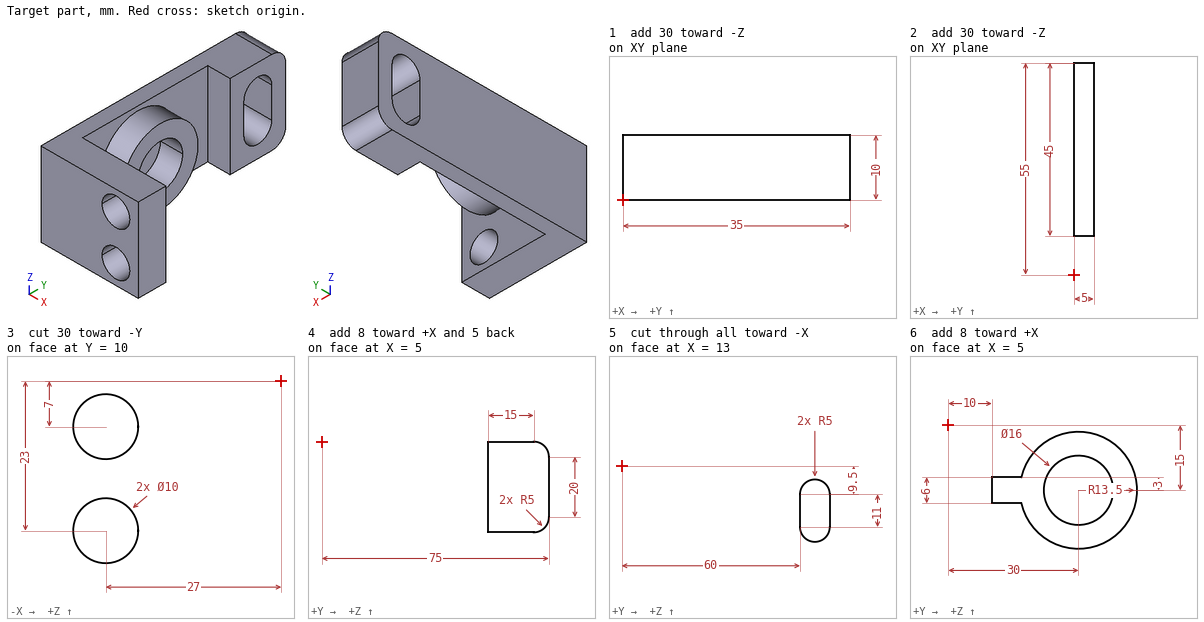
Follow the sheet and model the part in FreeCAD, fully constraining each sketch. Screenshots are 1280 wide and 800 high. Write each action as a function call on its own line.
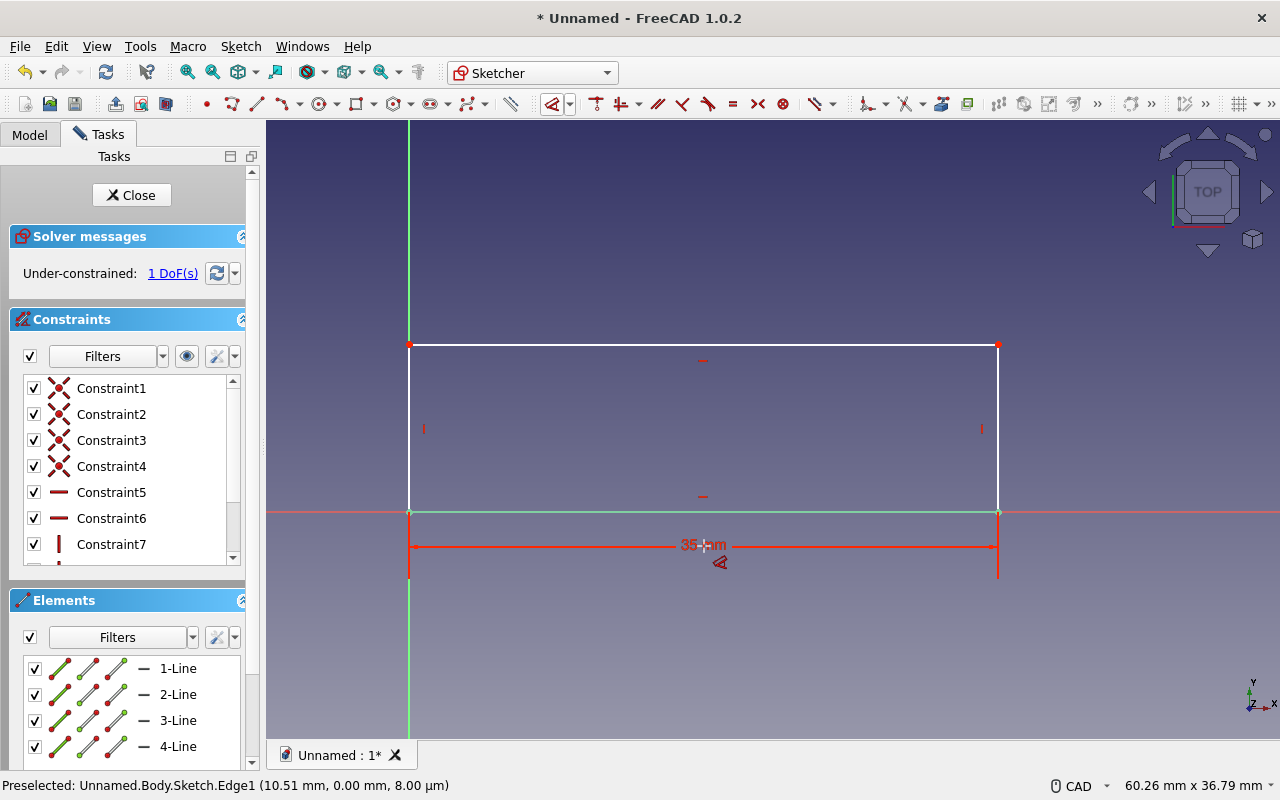
click(998, 462)
click(1032, 429)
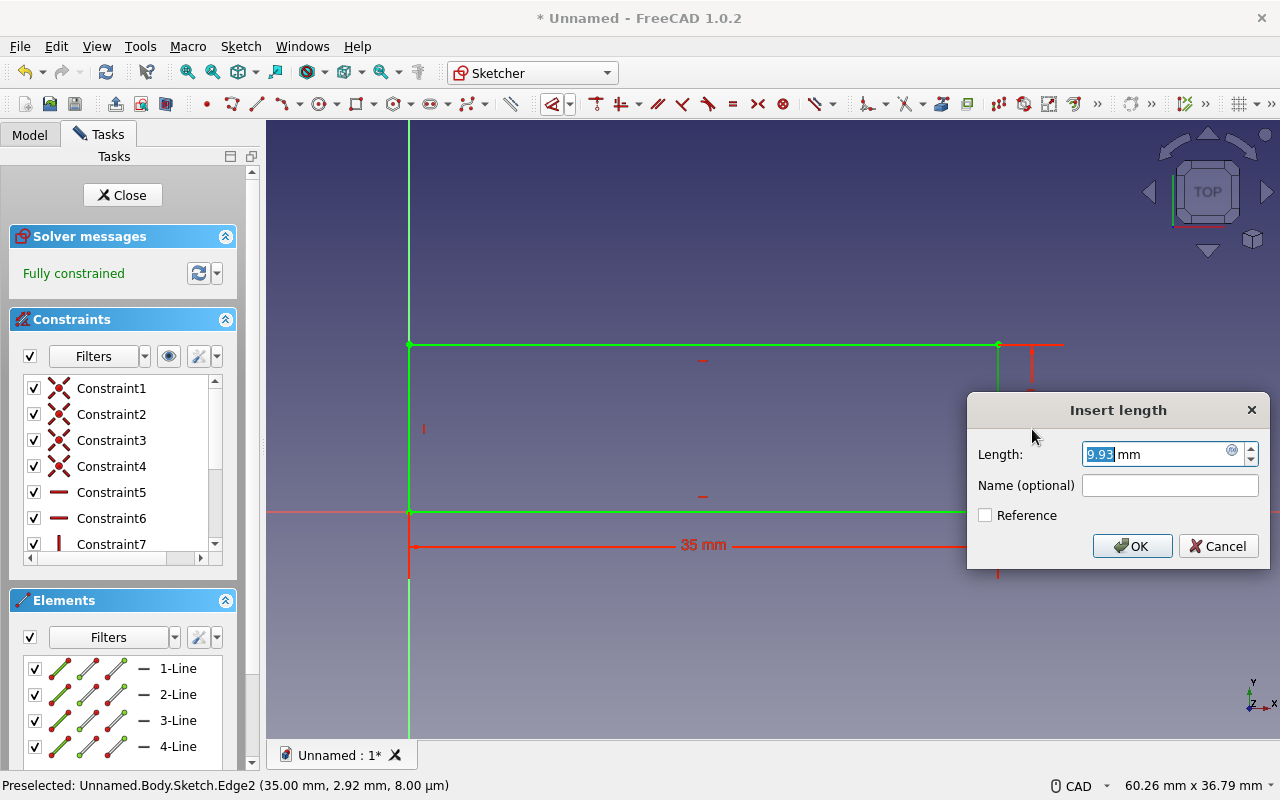
text(10)
key(Return)
key(Escape)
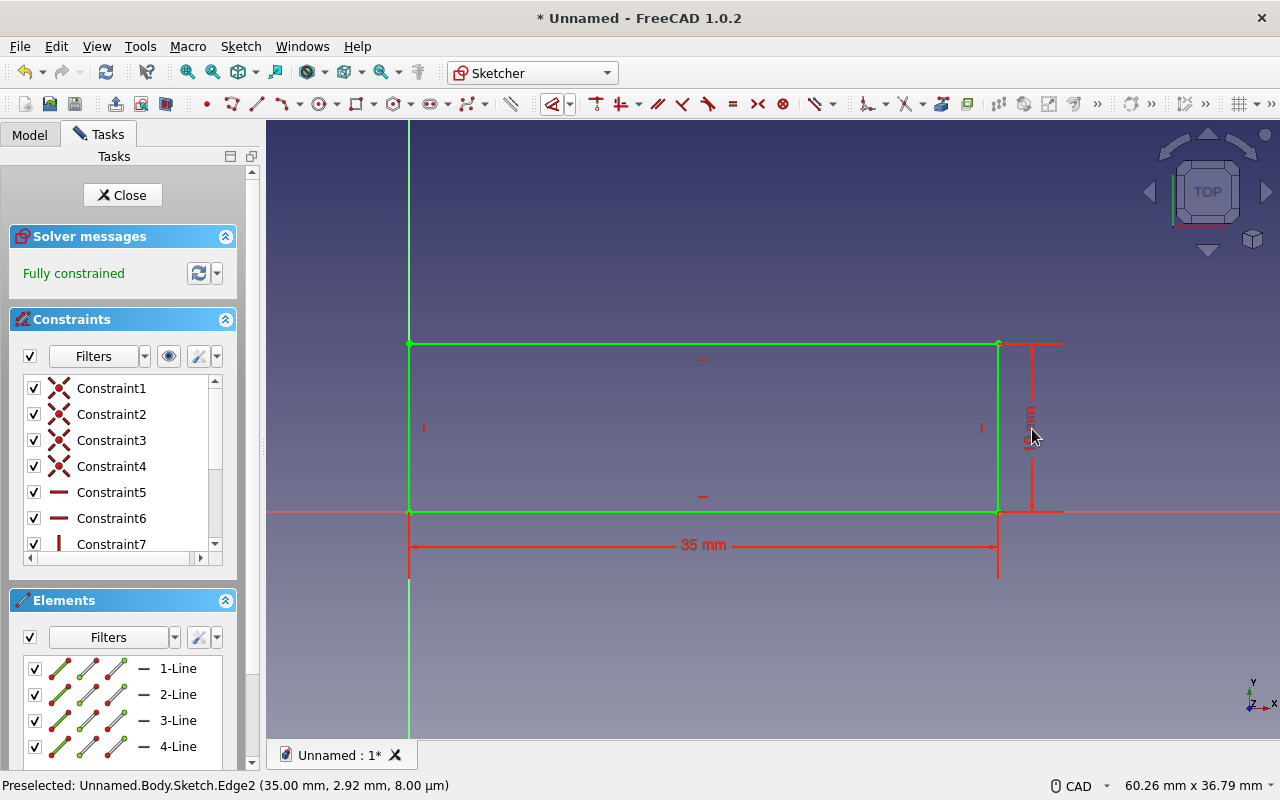
click(123, 195)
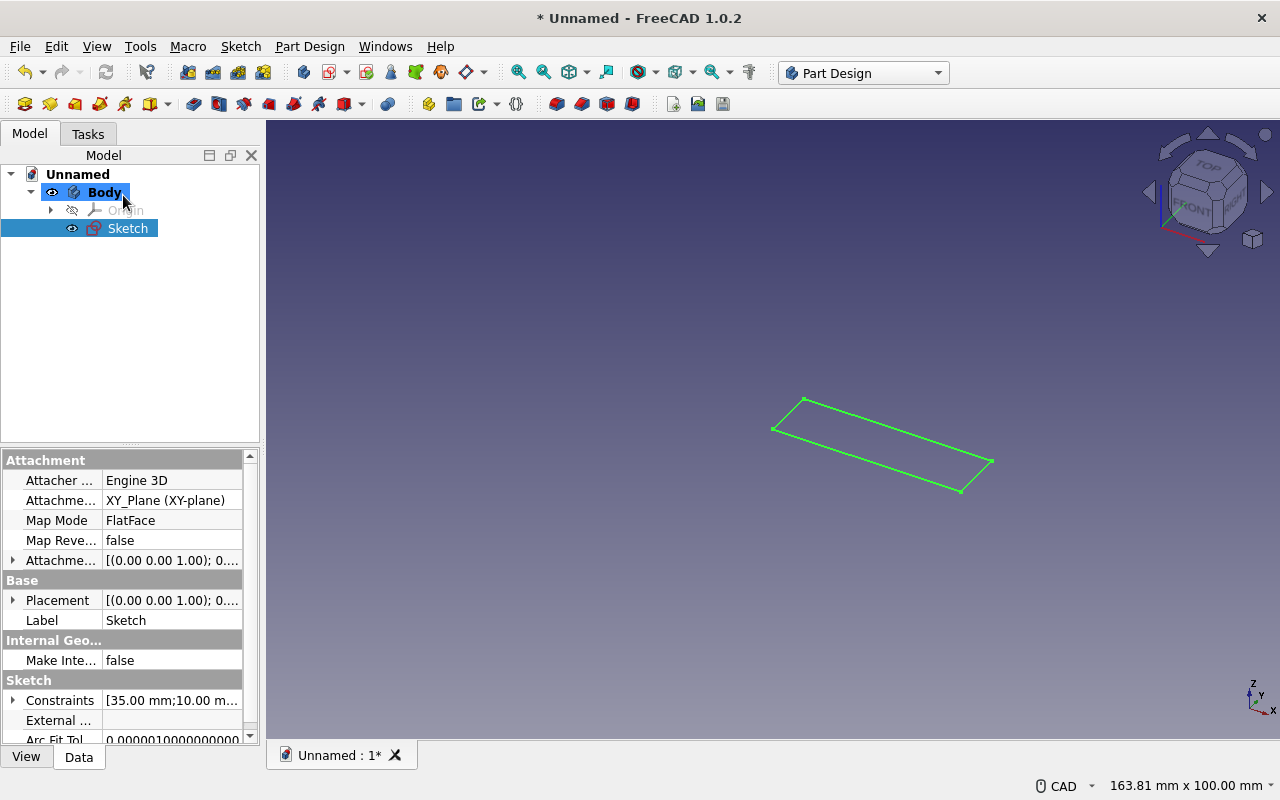
click(25, 104)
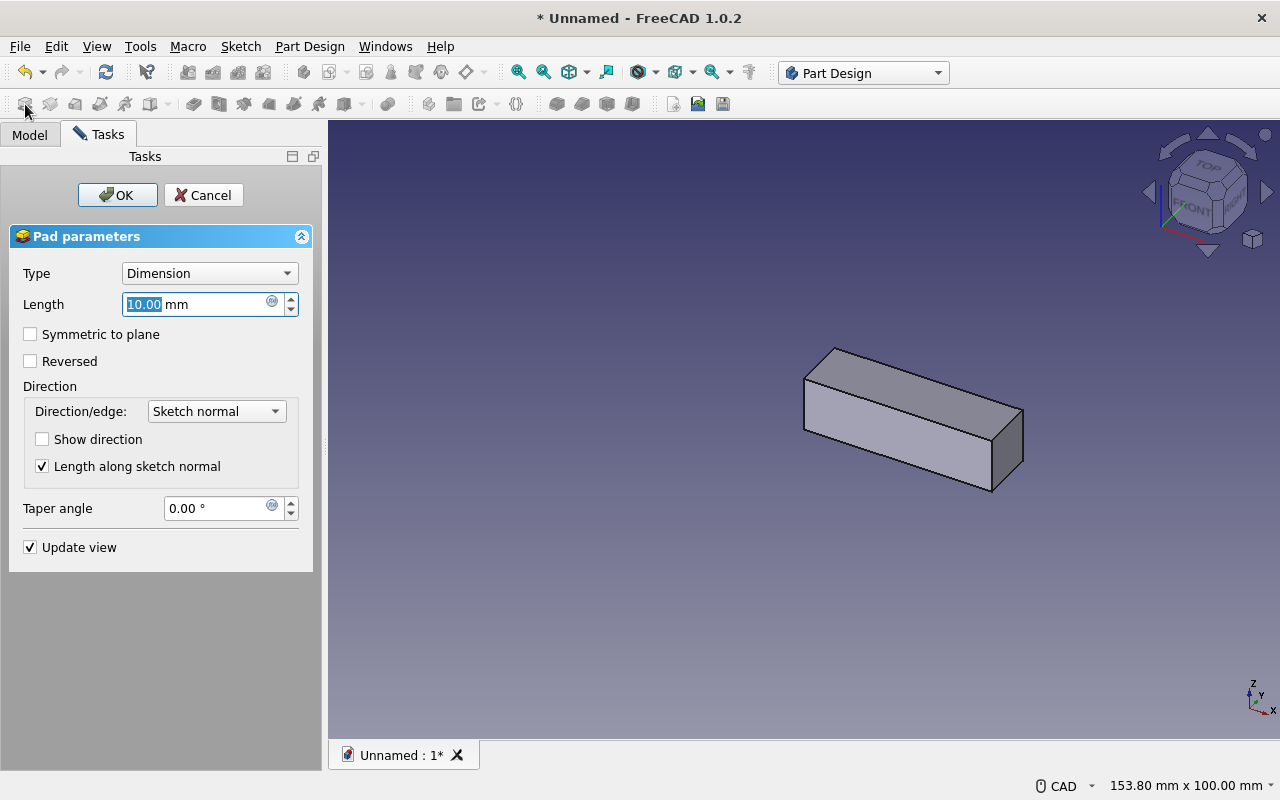
text(30)
key(Tab)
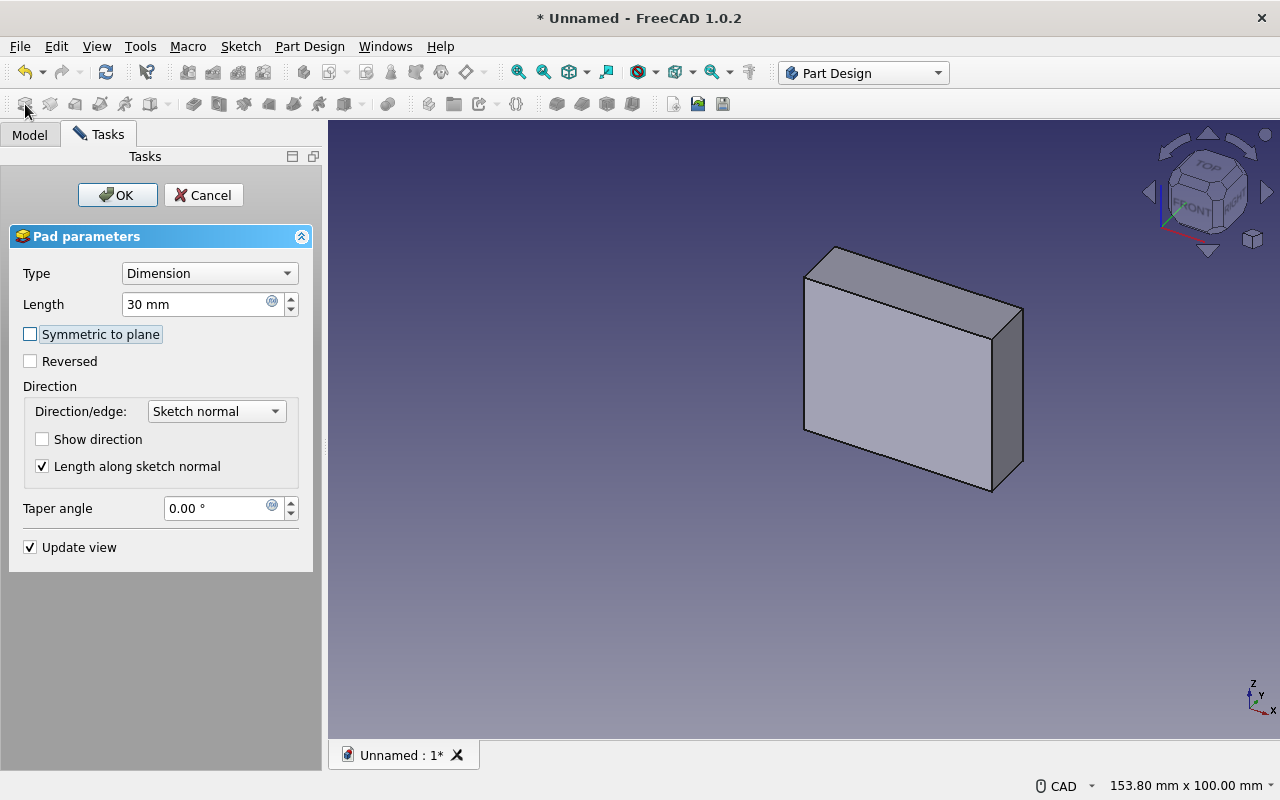
click(31, 361)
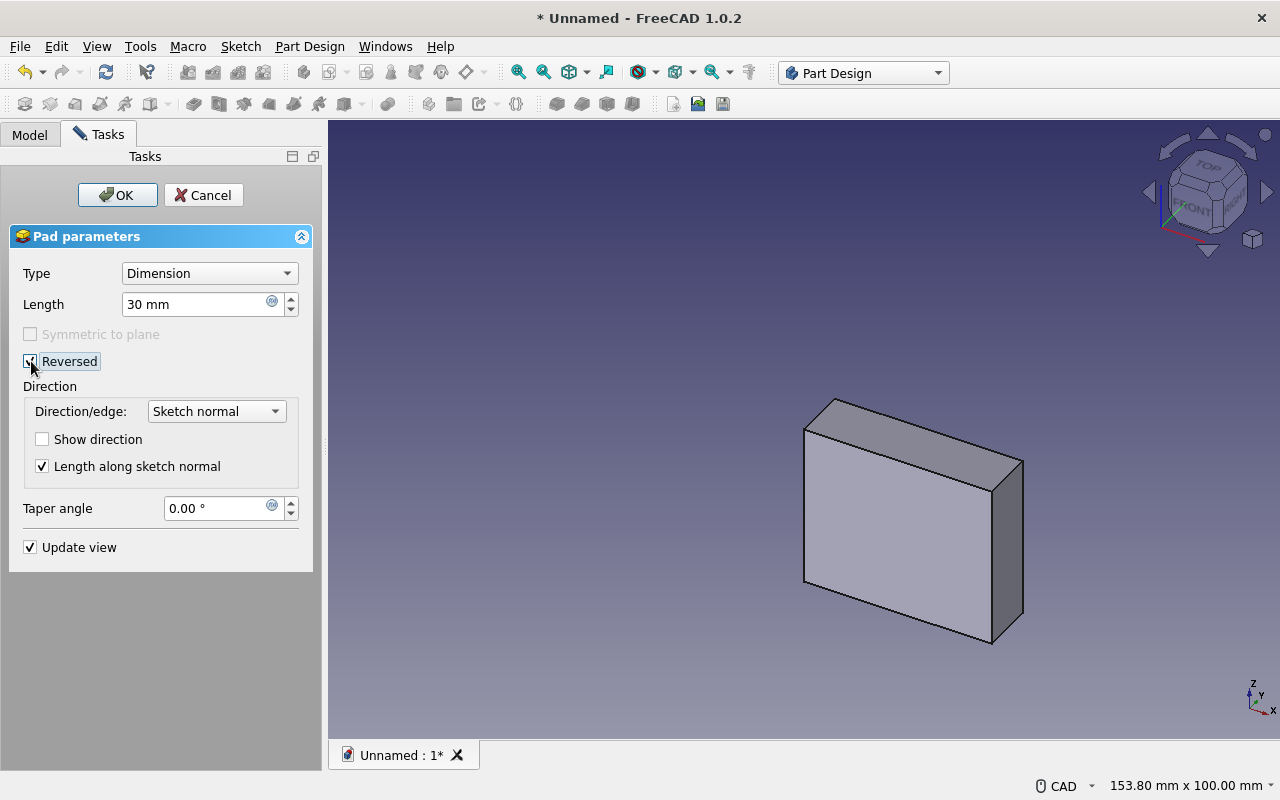
click(118, 195)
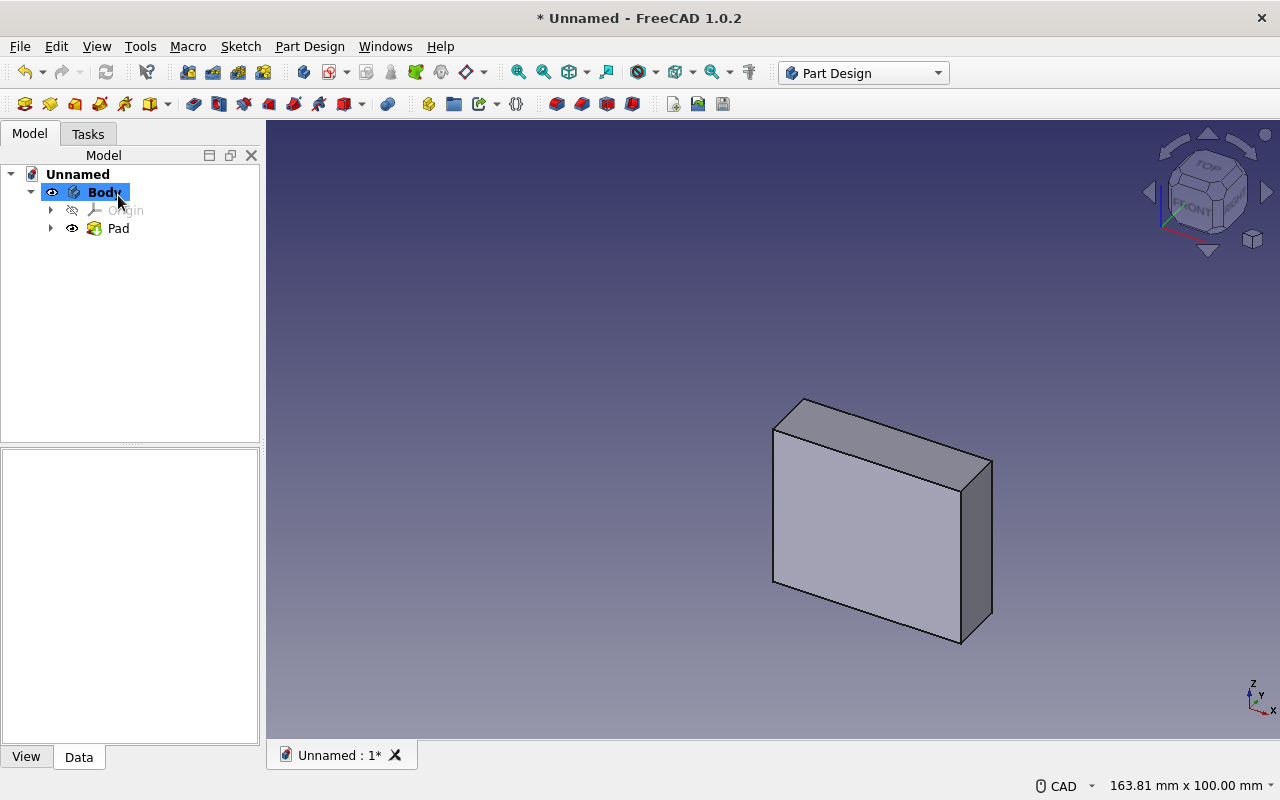
click(519, 72)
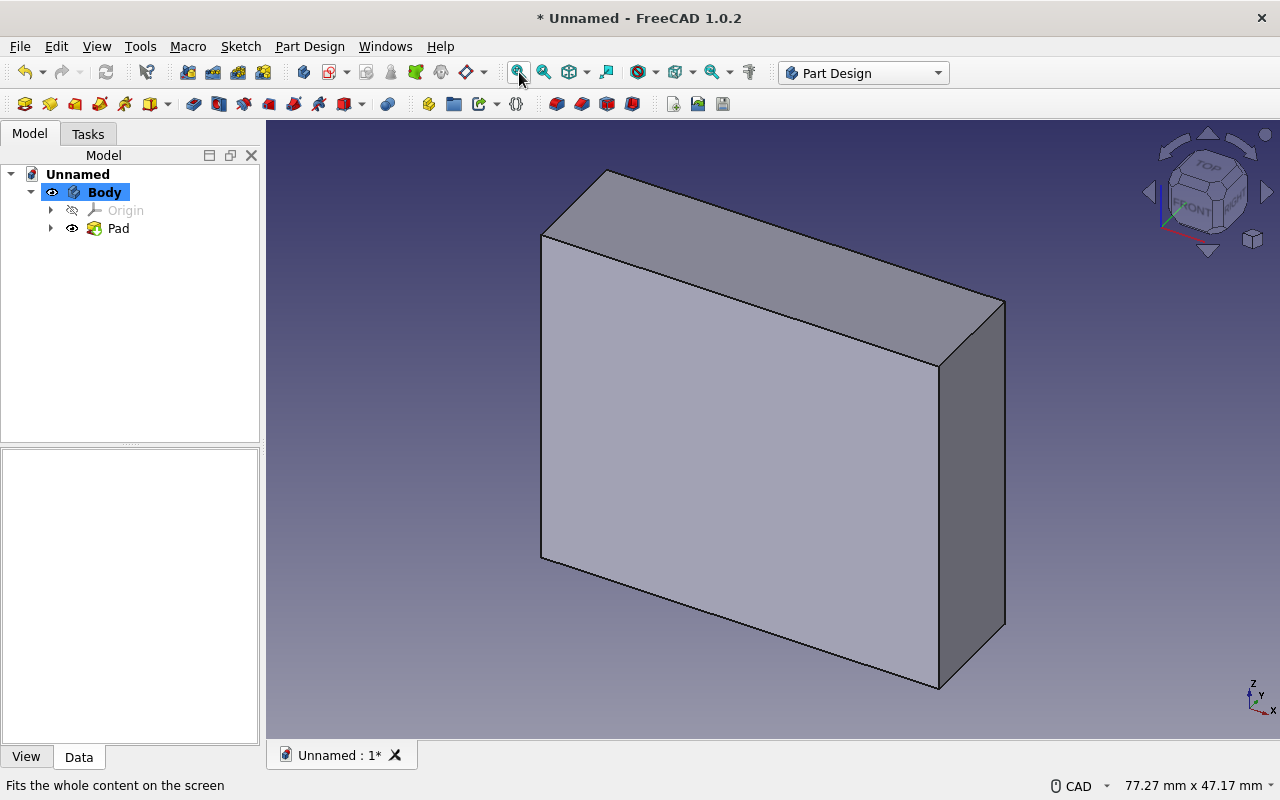
click(328, 72)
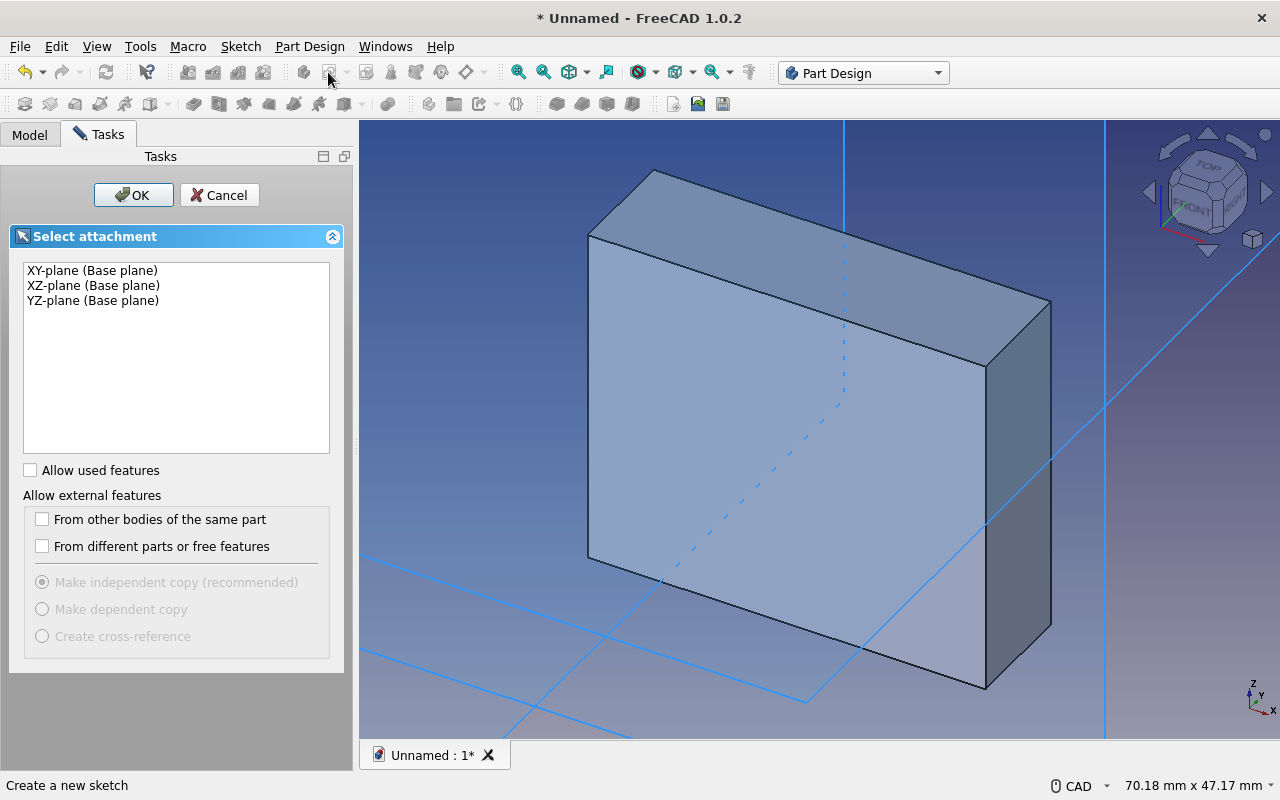
click(84, 270)